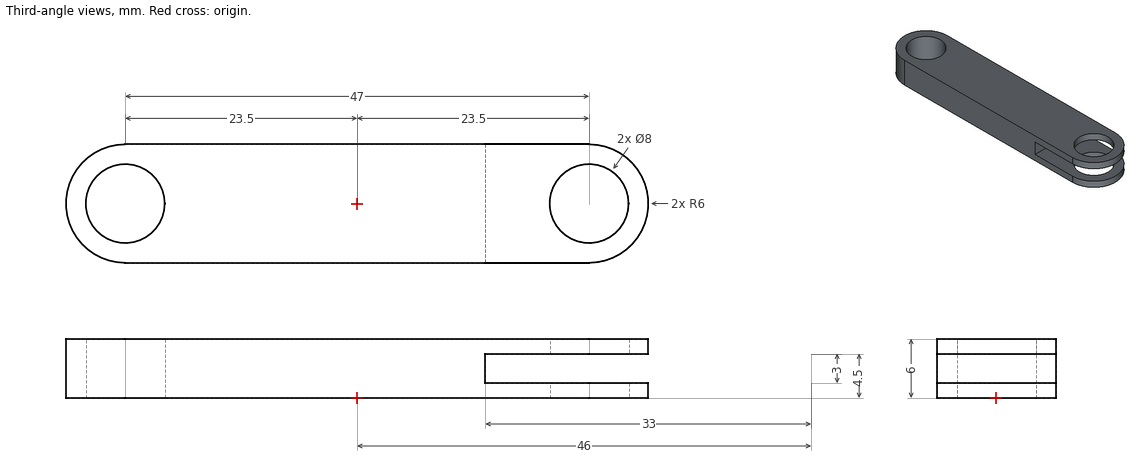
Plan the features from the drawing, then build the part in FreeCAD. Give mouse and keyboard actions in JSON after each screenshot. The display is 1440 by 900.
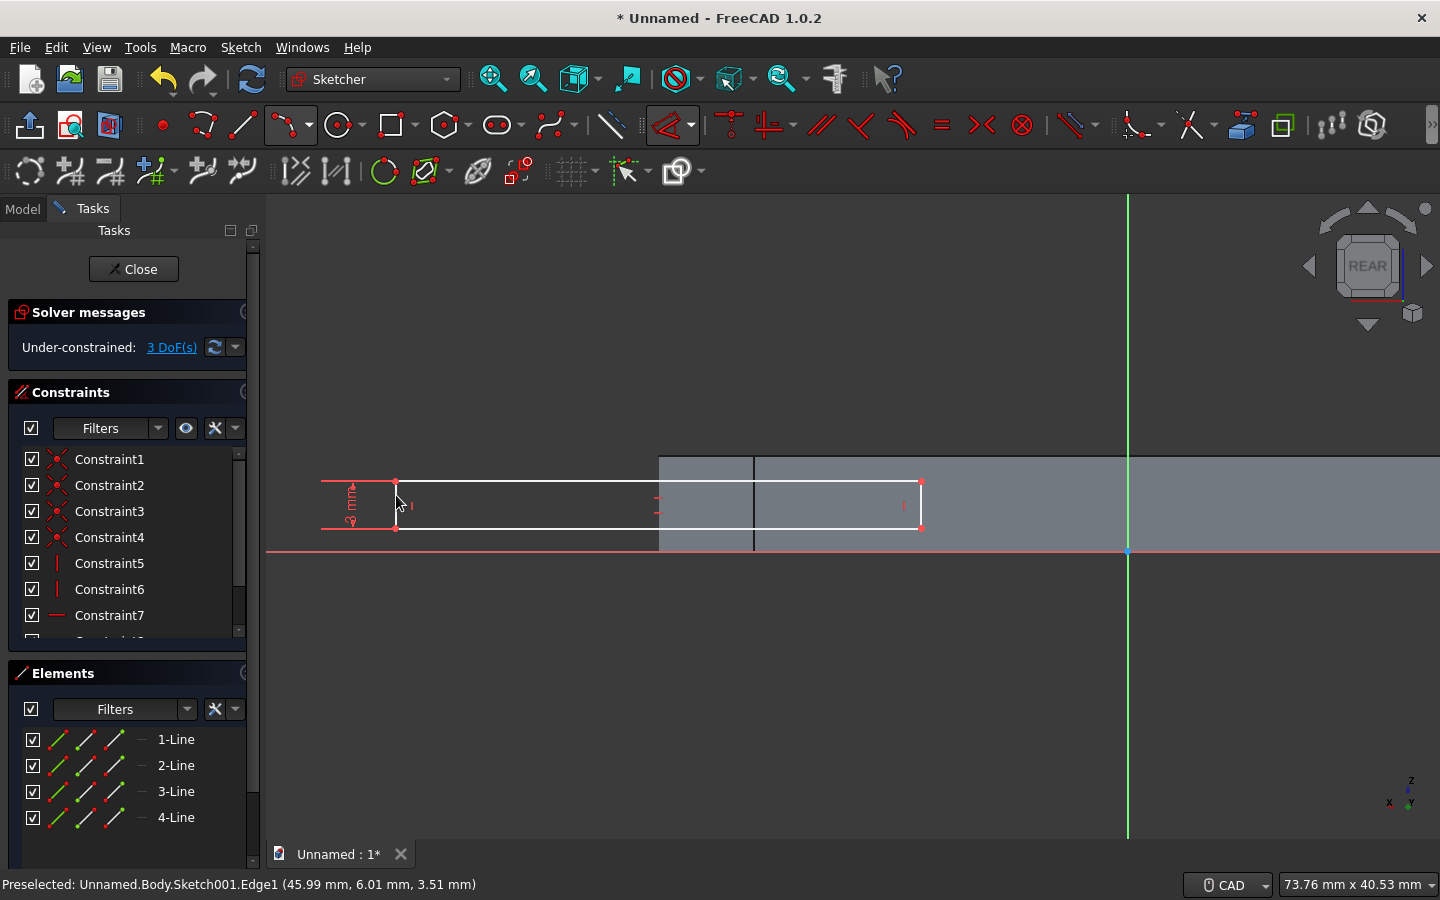
{"action": "left_click", "coordinate": [554, 529]}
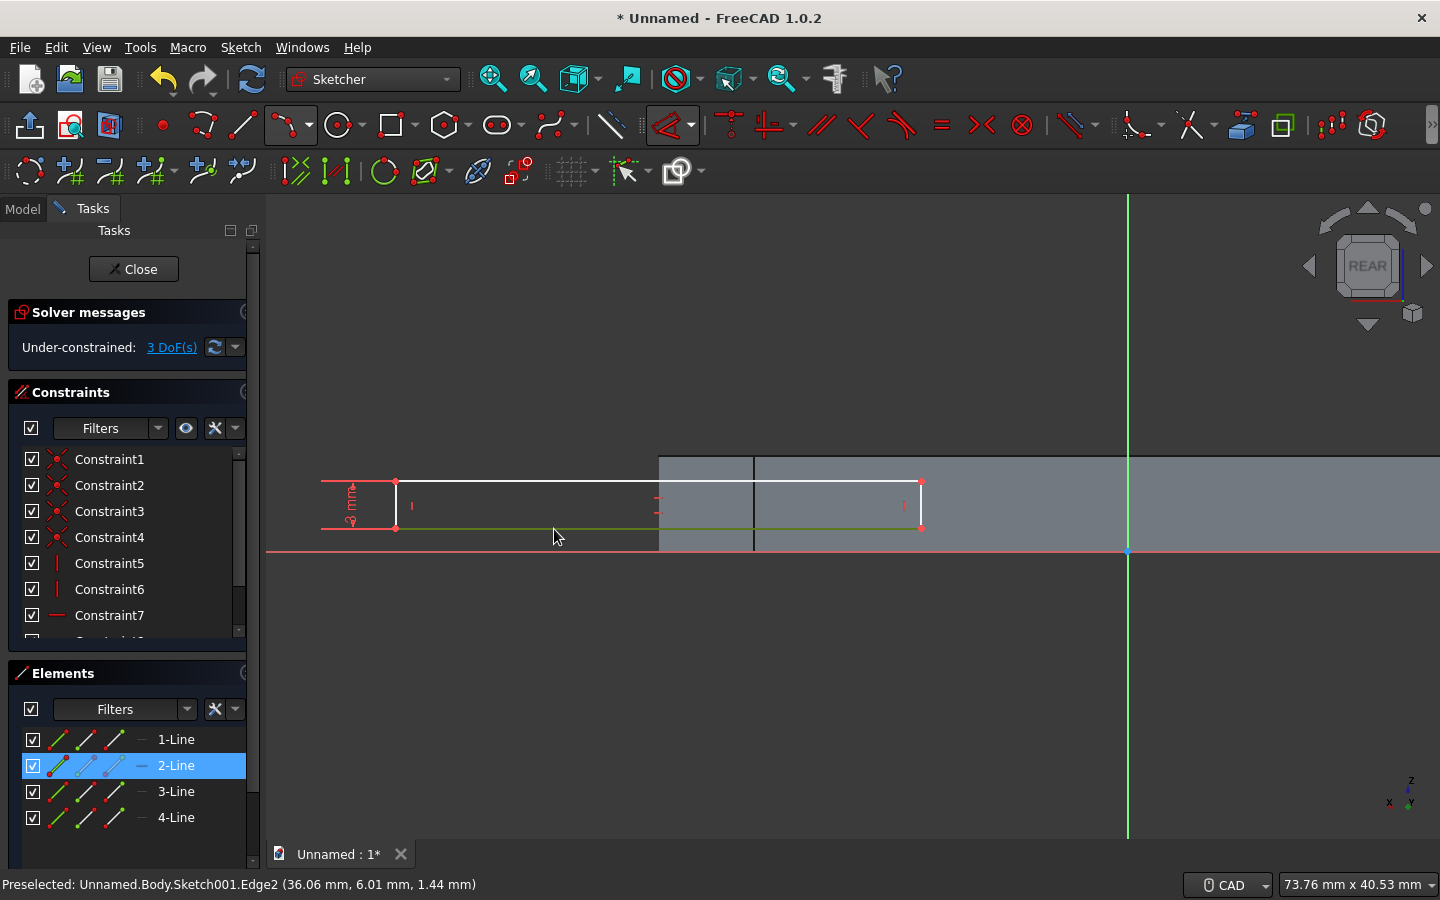
{"action": "key", "text": "l"}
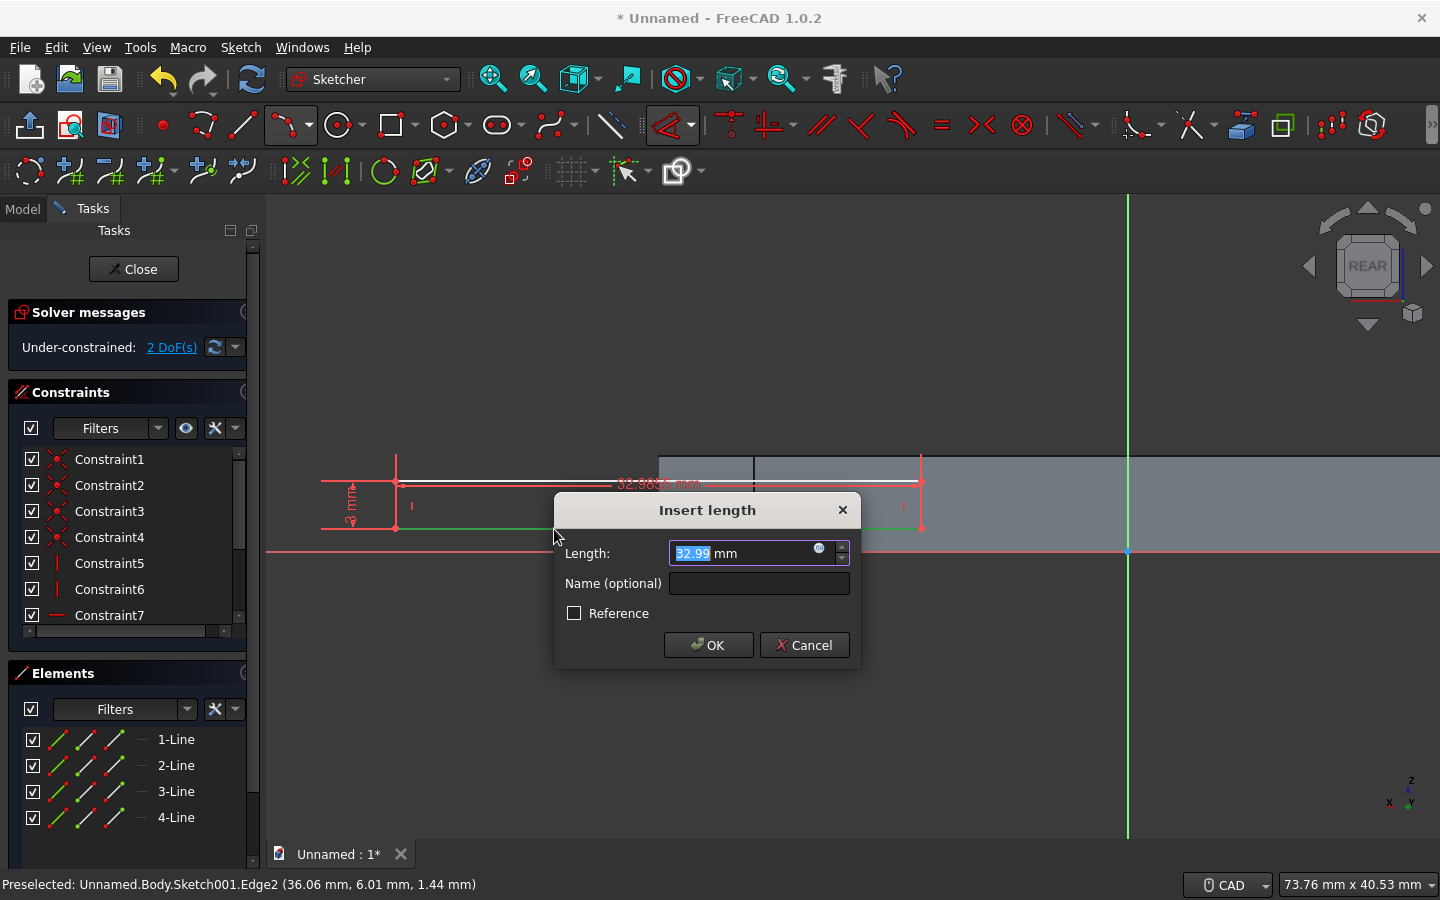
{"action": "type", "text": "33"}
{"action": "key", "text": "Return"}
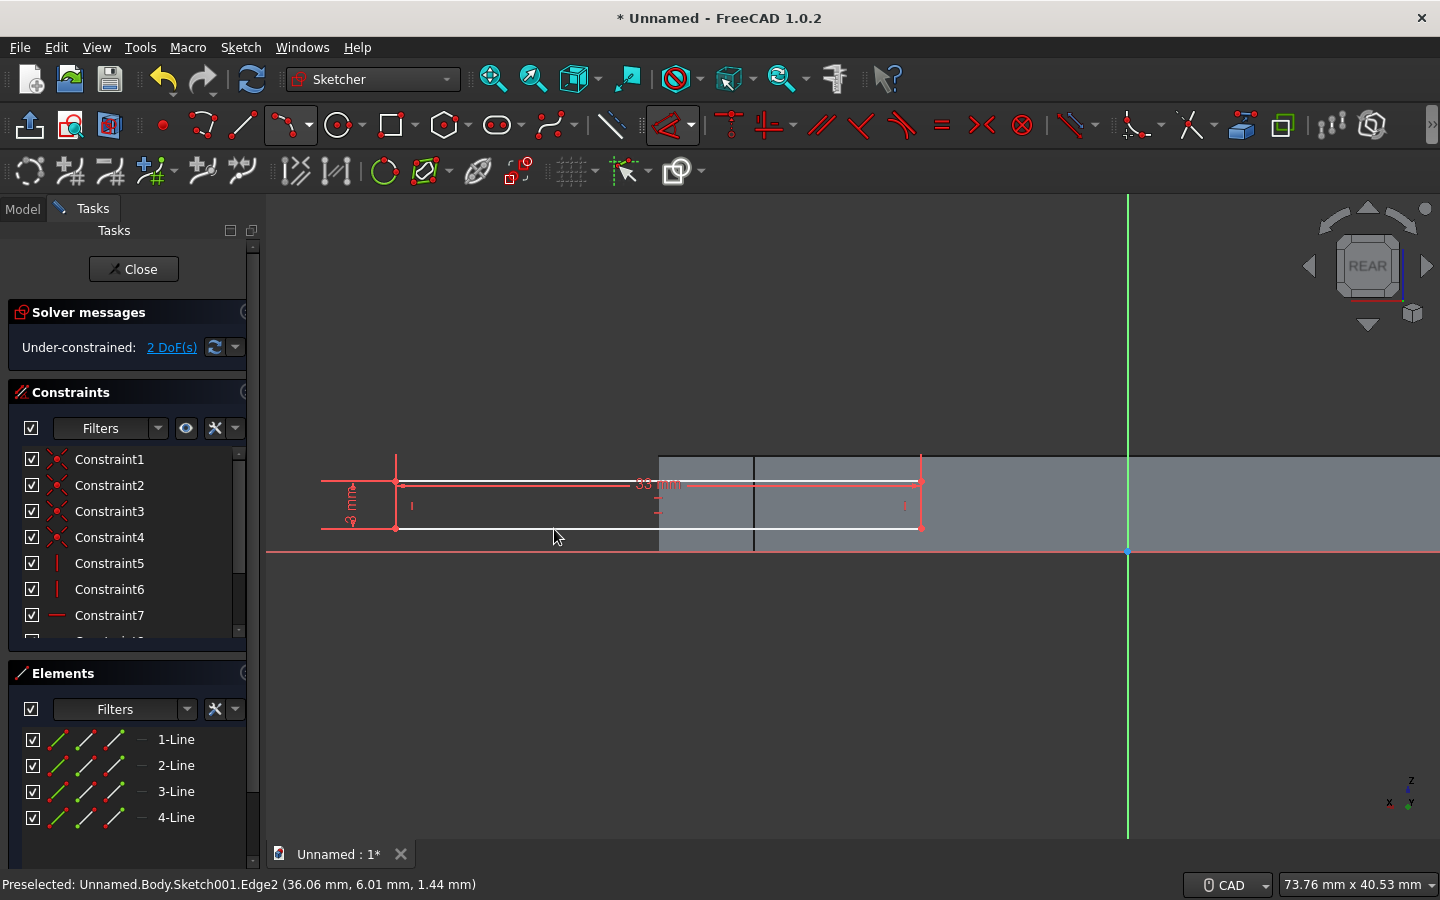
{"action": "left_click", "coordinate": [396, 481]}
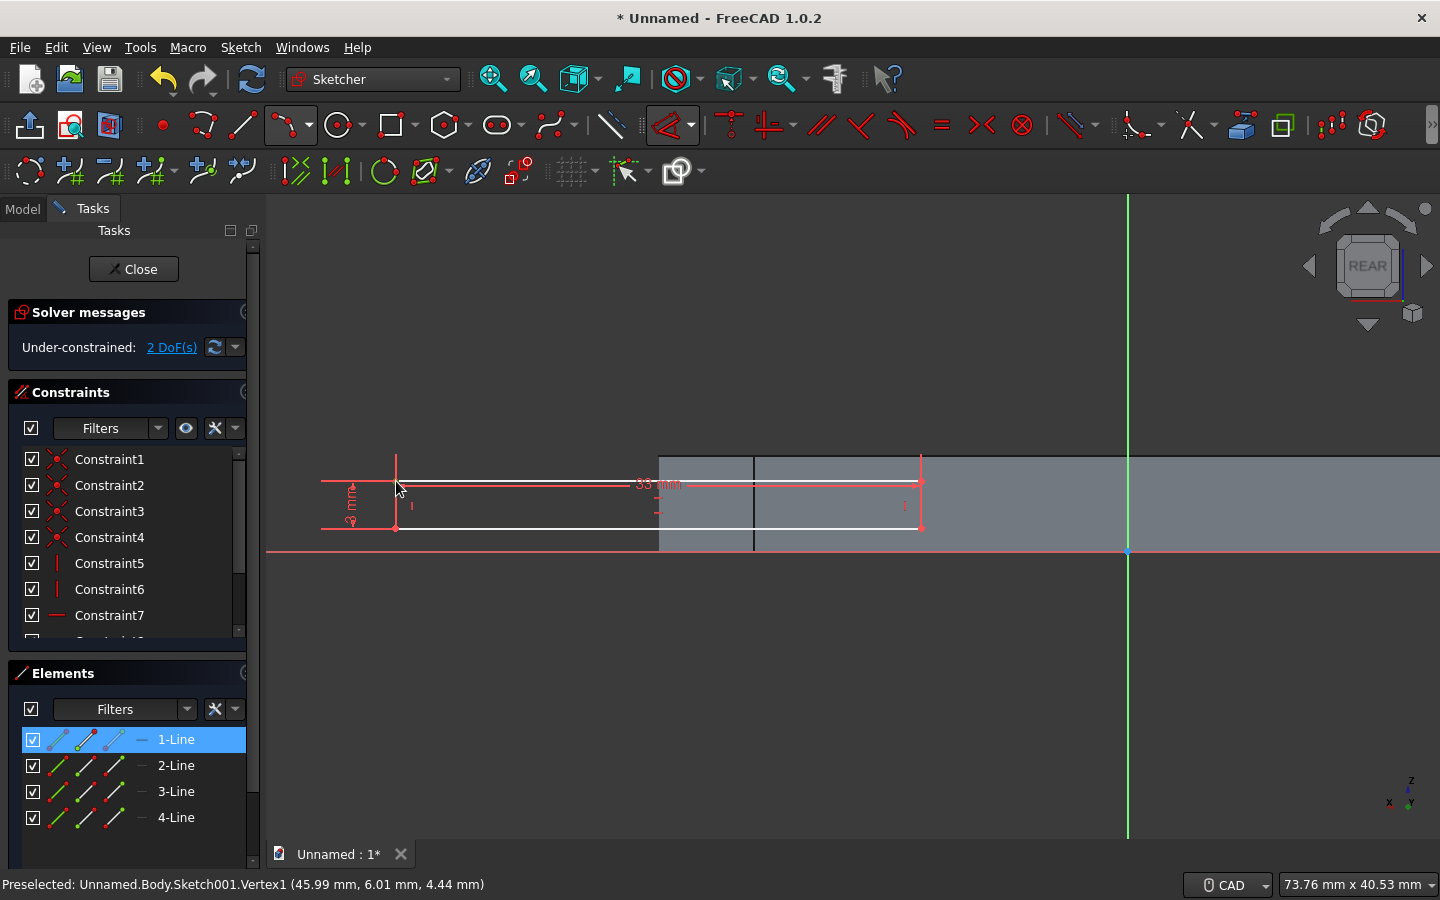
{"action": "key", "text": "l"}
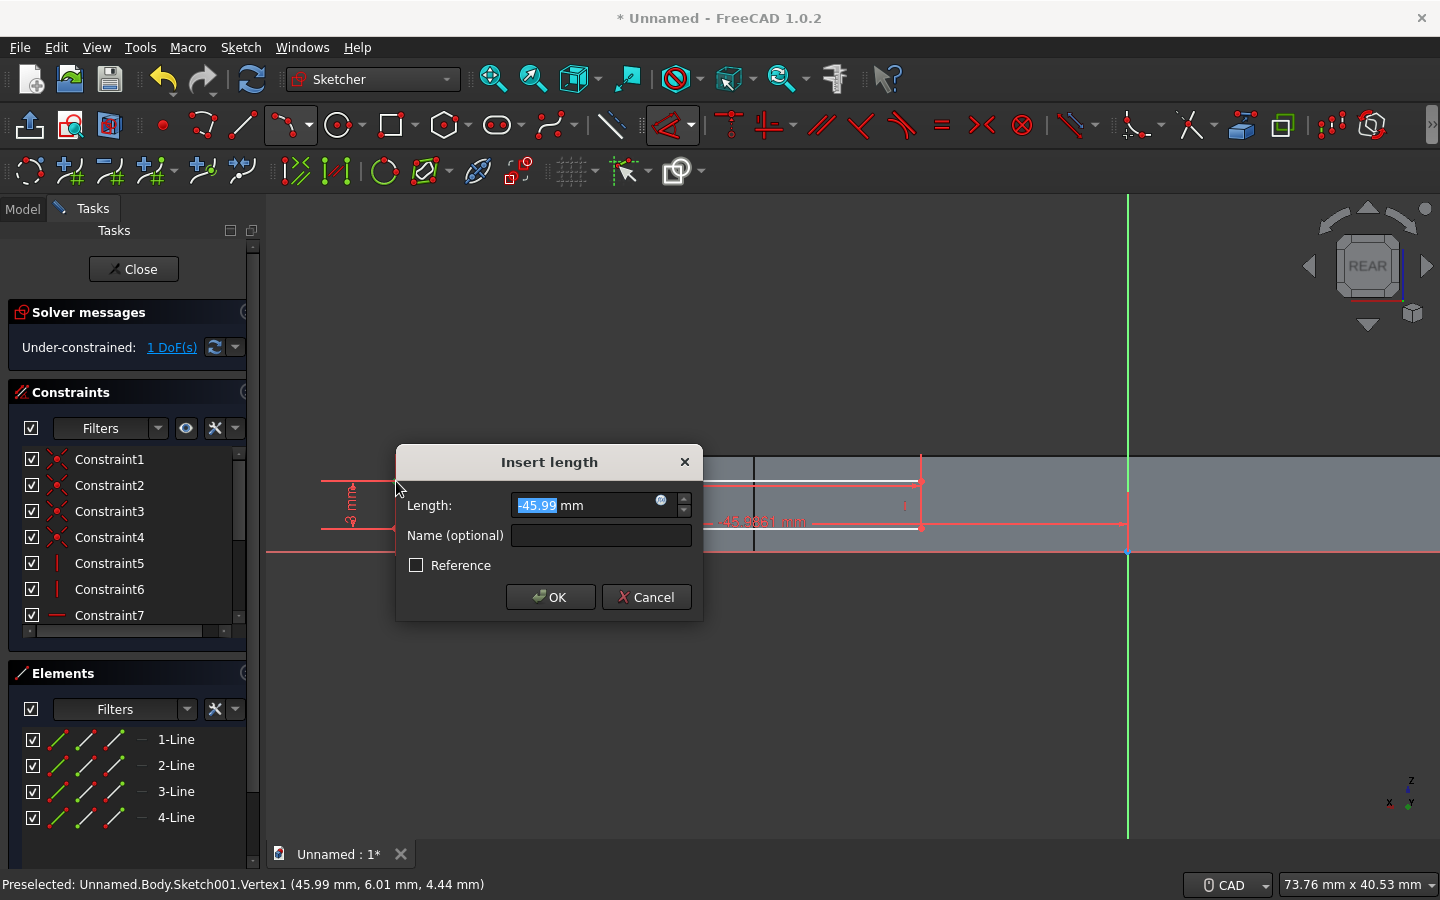
{"action": "type", "text": "-46"}
{"action": "key", "text": "Return"}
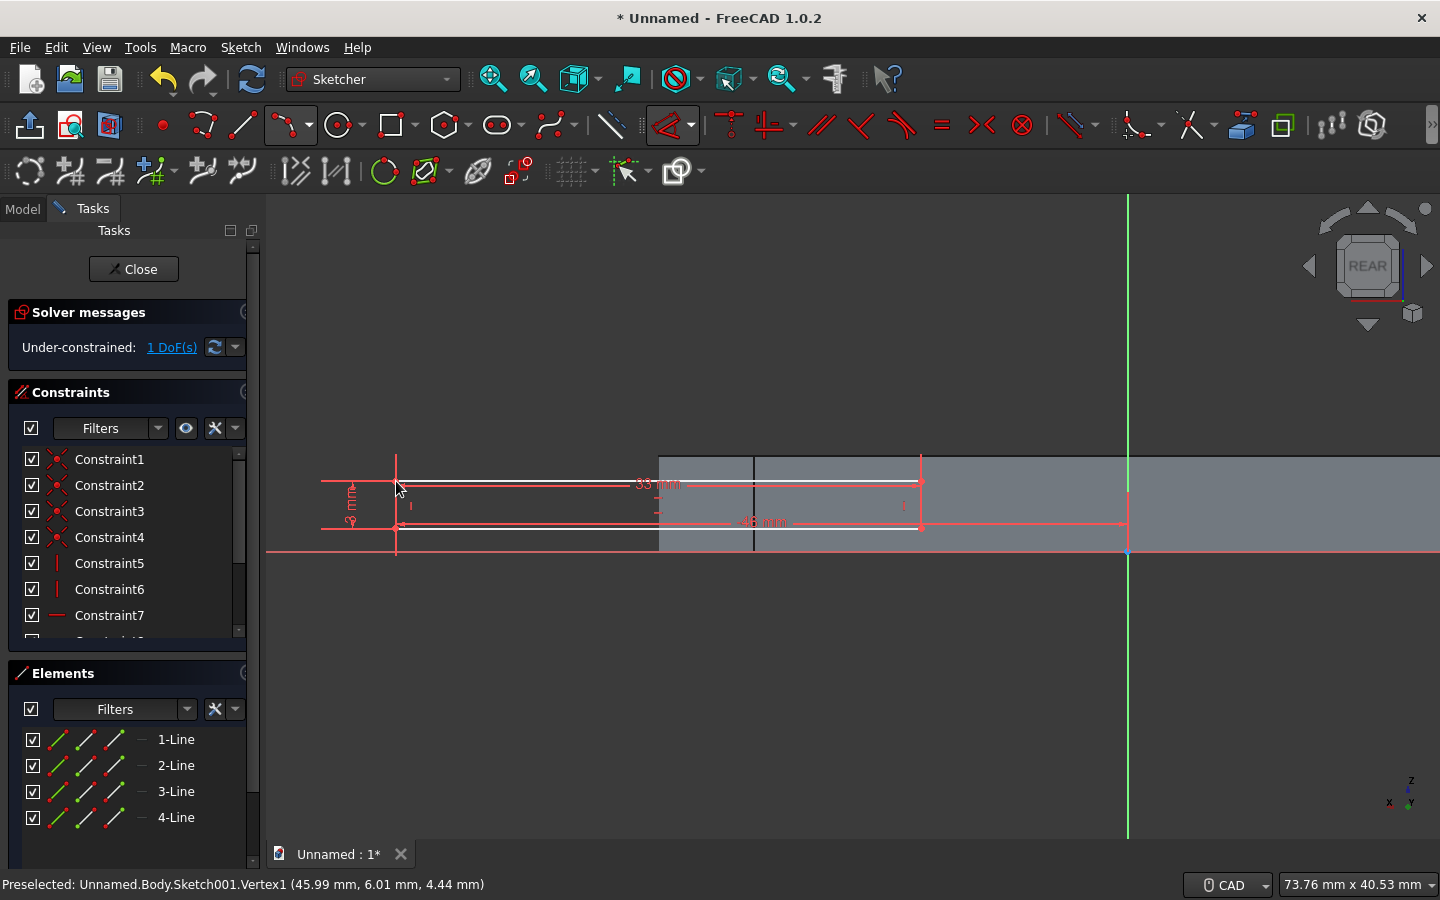
{"action": "left_click", "coordinate": [396, 481]}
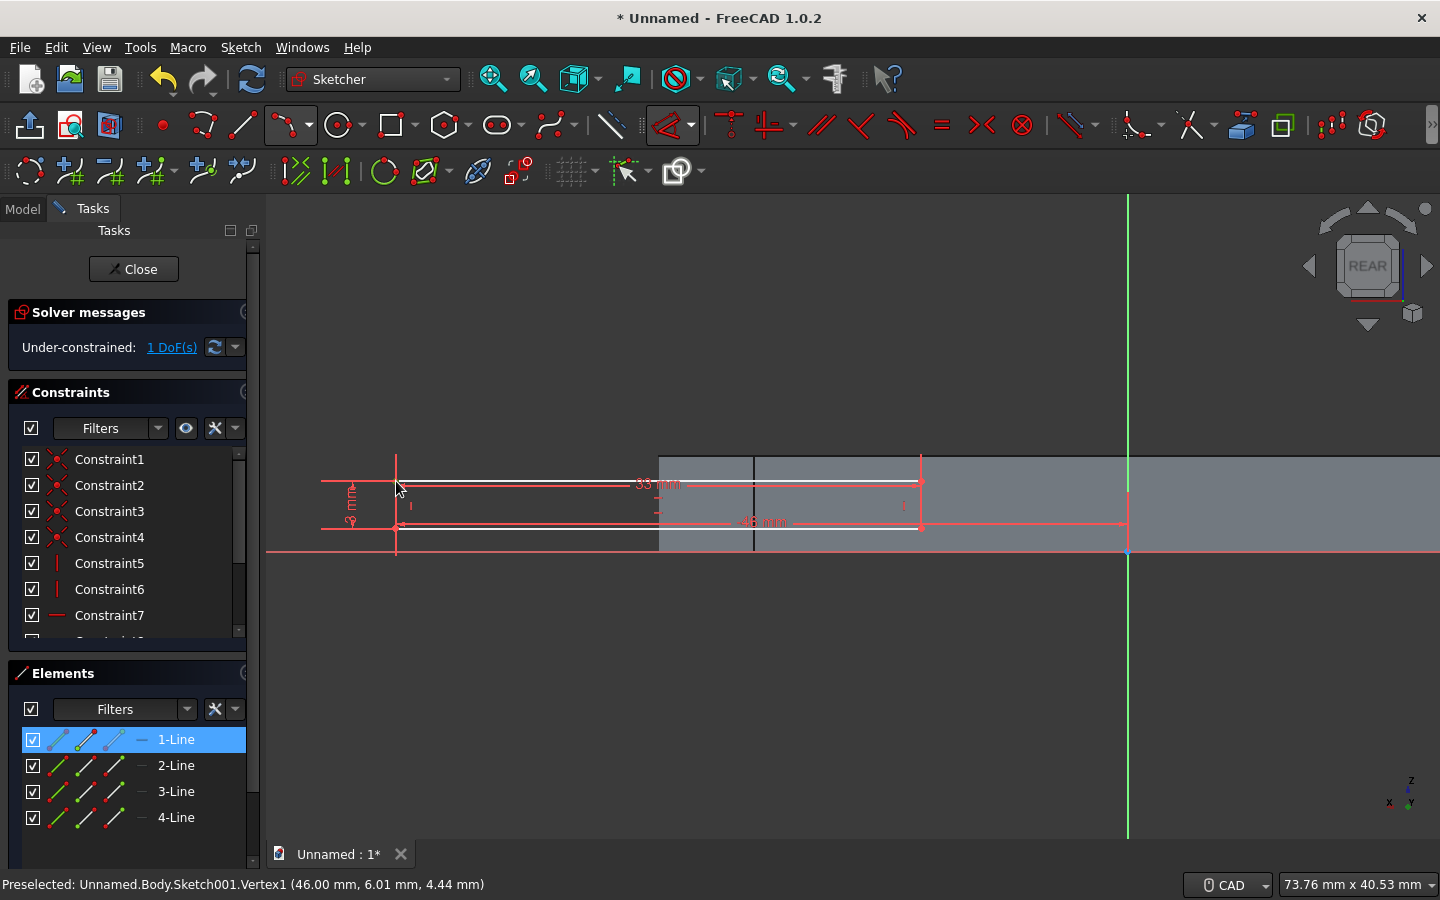
{"action": "key", "text": "i"}